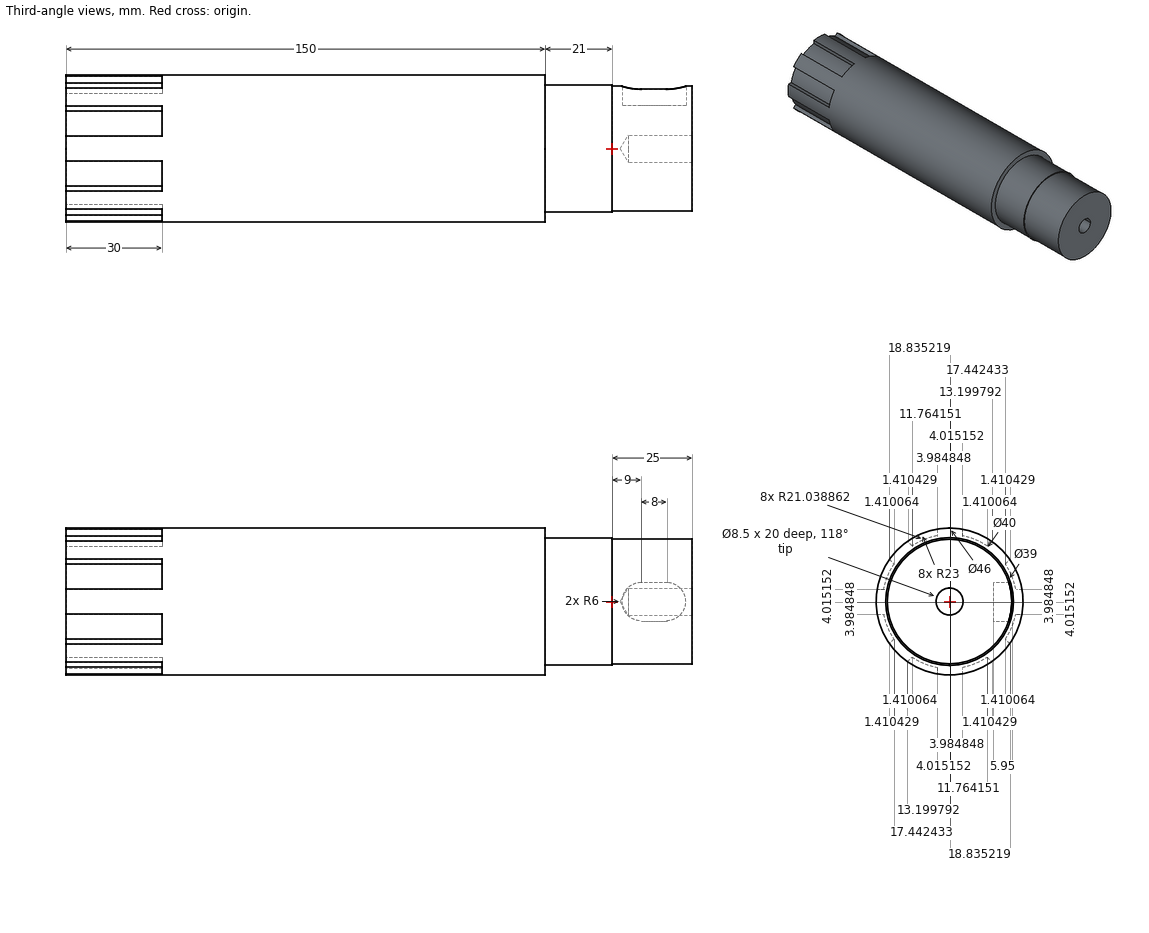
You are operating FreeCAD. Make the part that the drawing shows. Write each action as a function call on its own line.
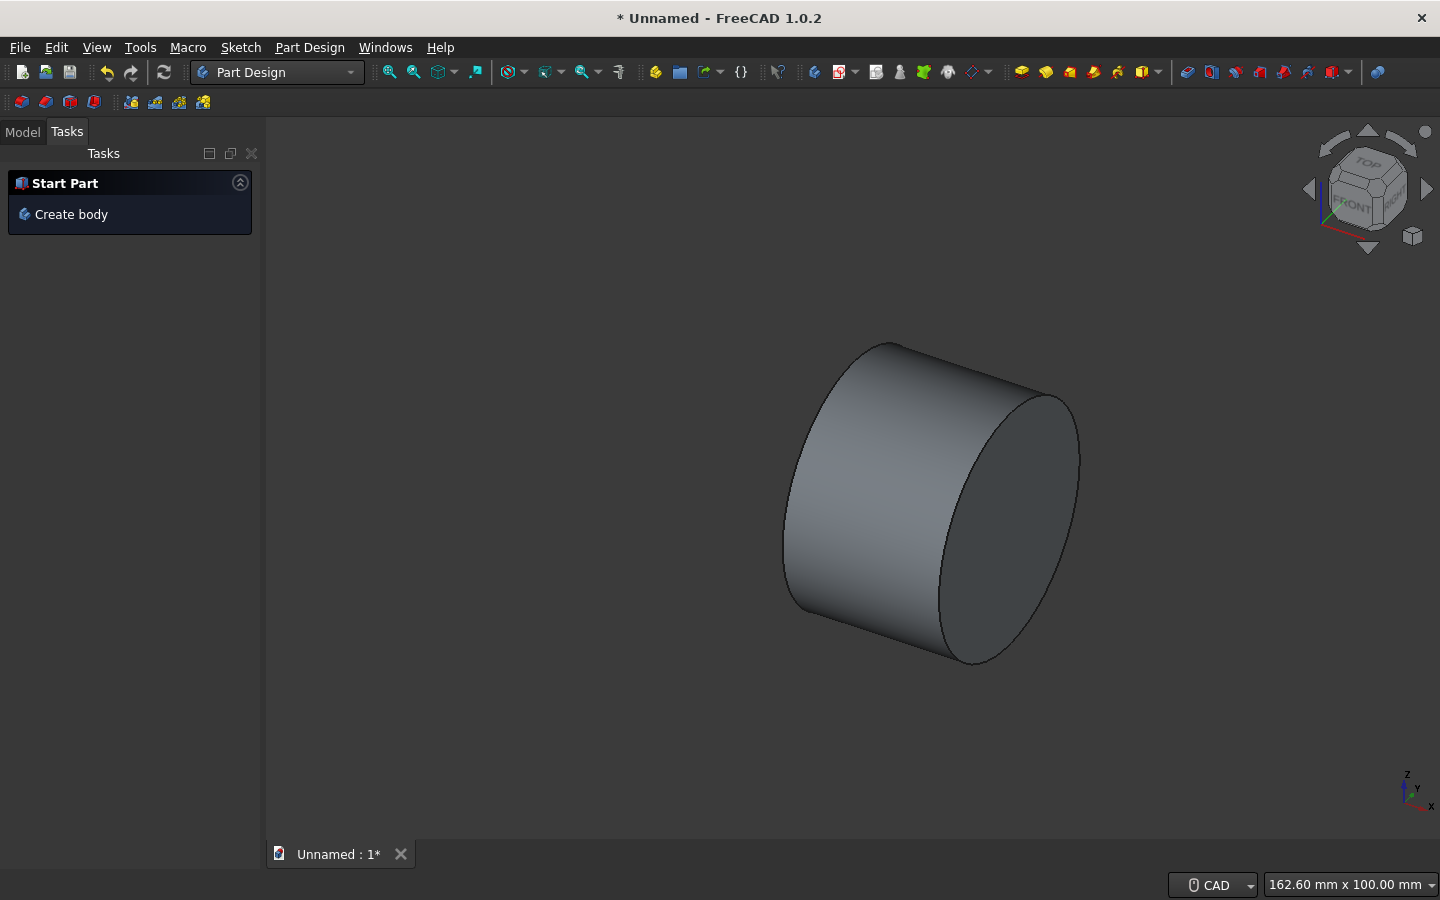
click(23, 131)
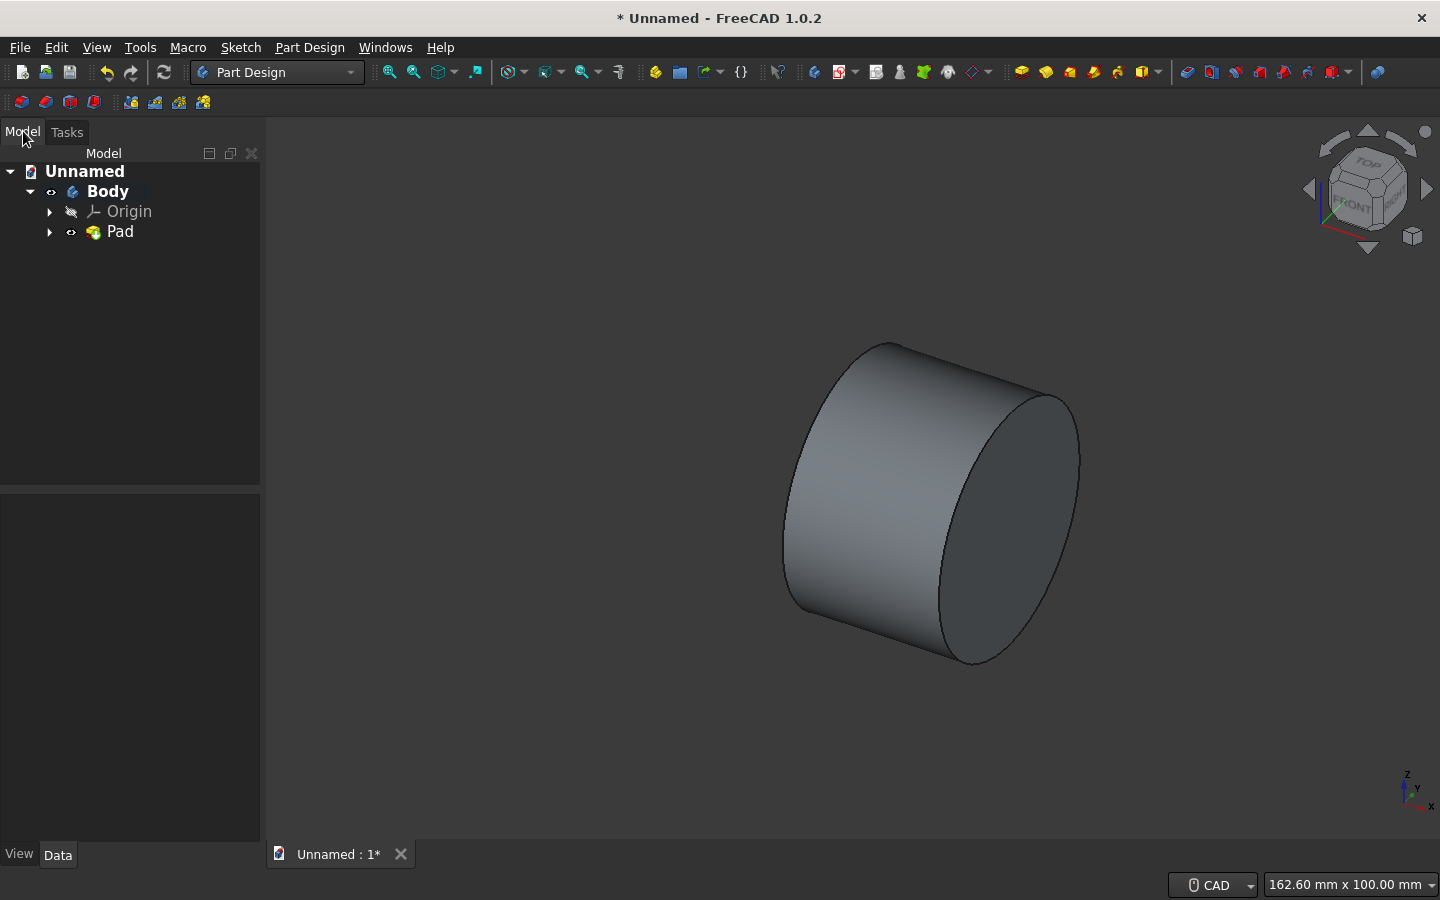
click(50, 212)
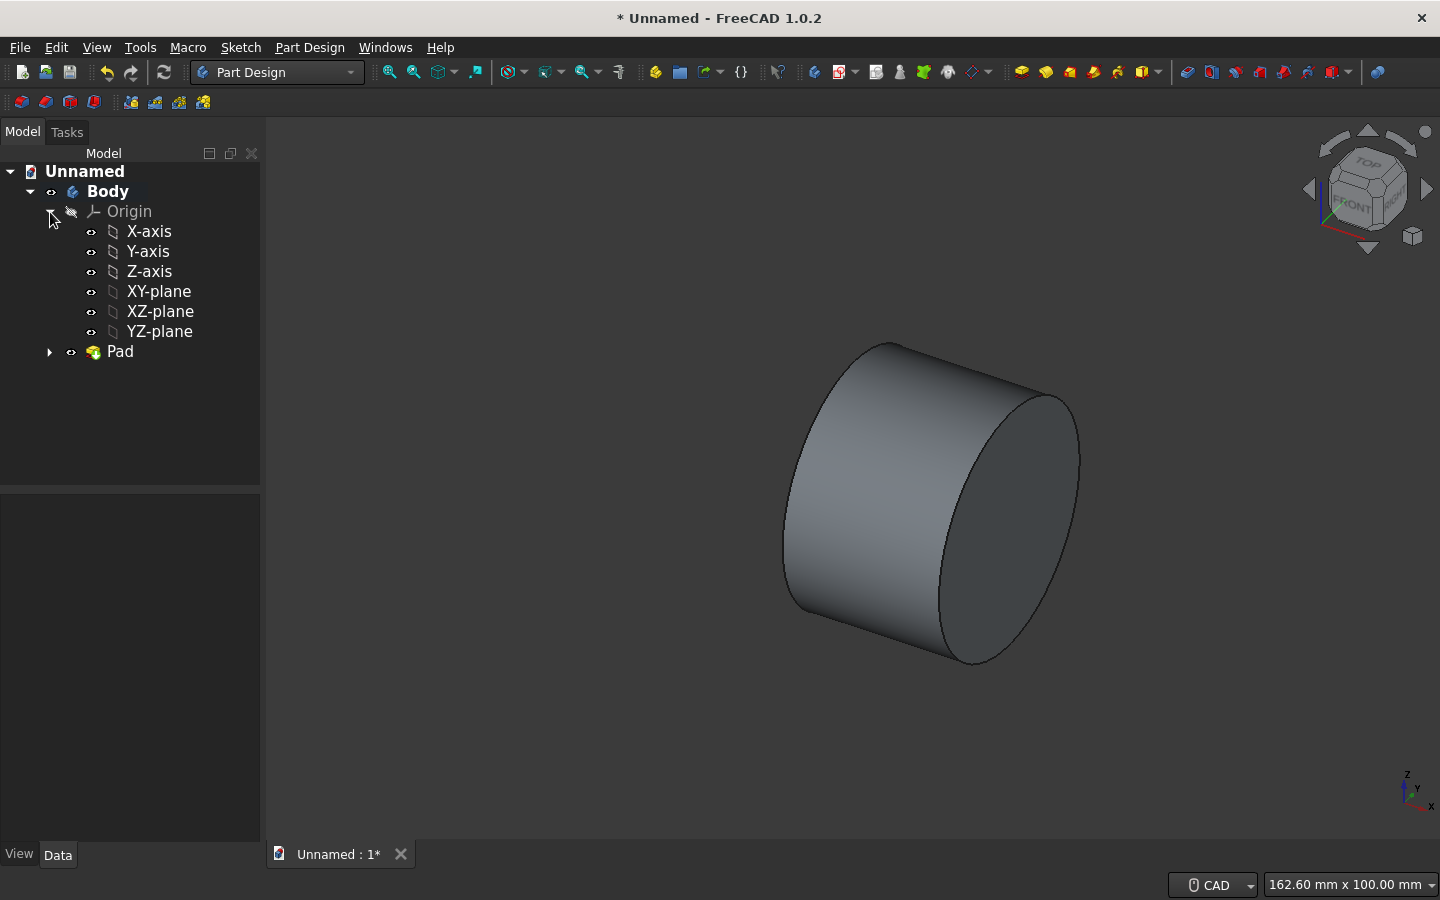
click(136, 312)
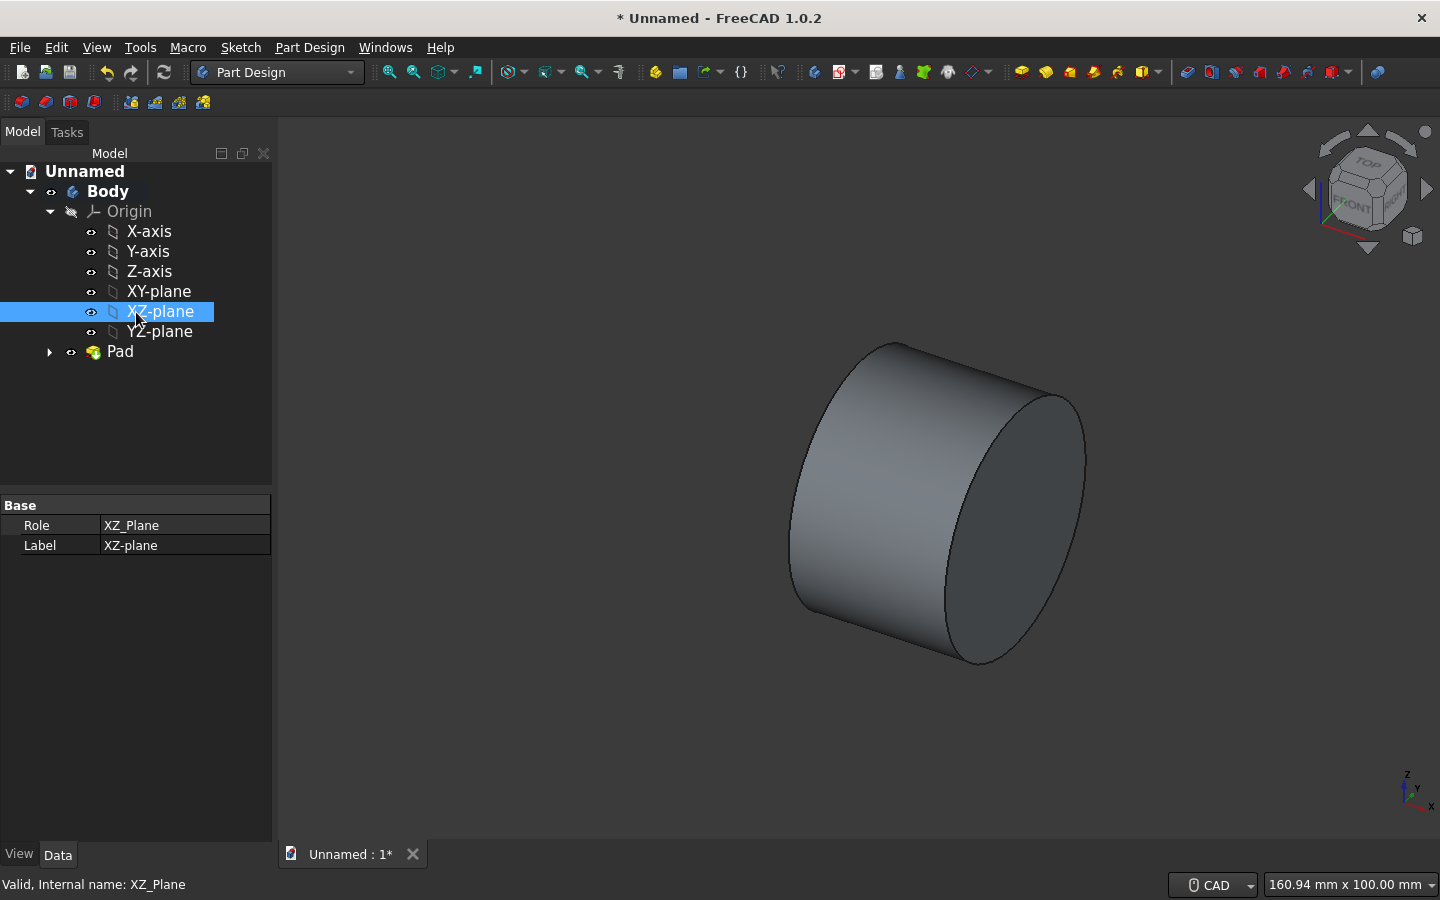
click(972, 72)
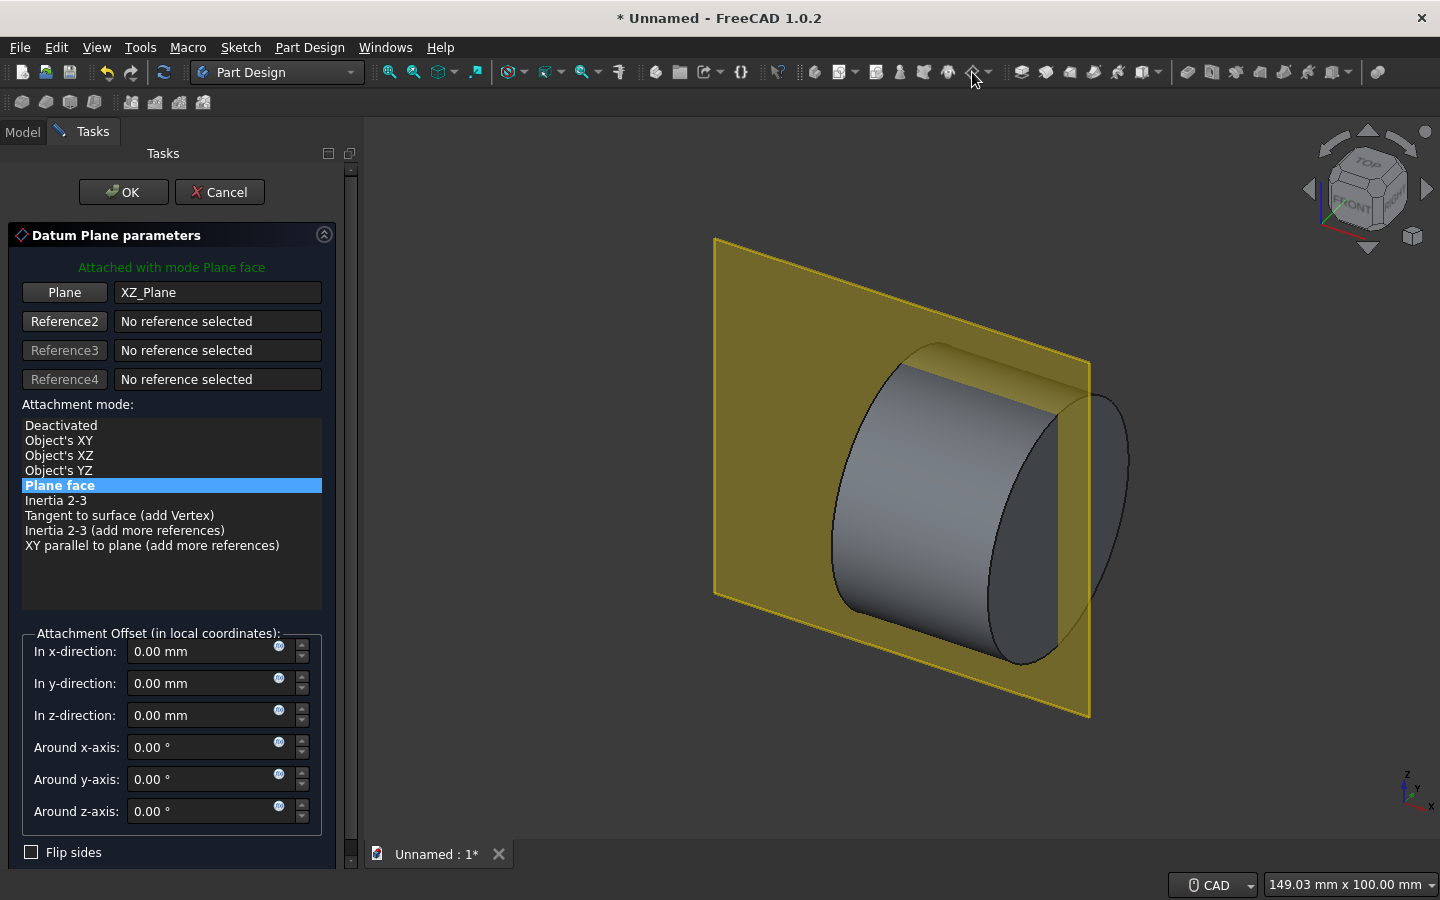
triple_click(210, 715)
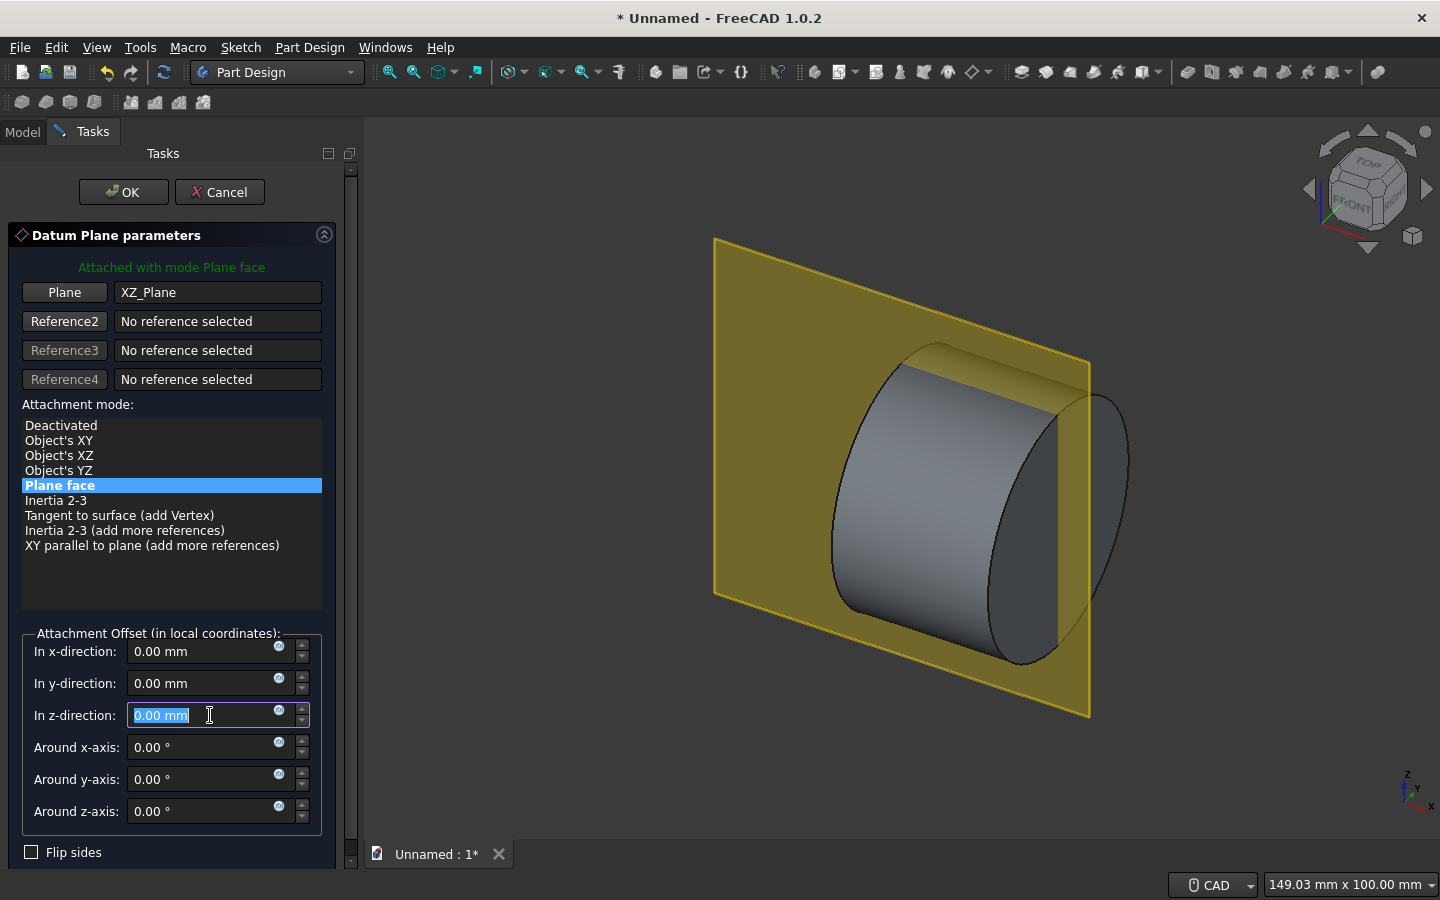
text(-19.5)
key(Tab)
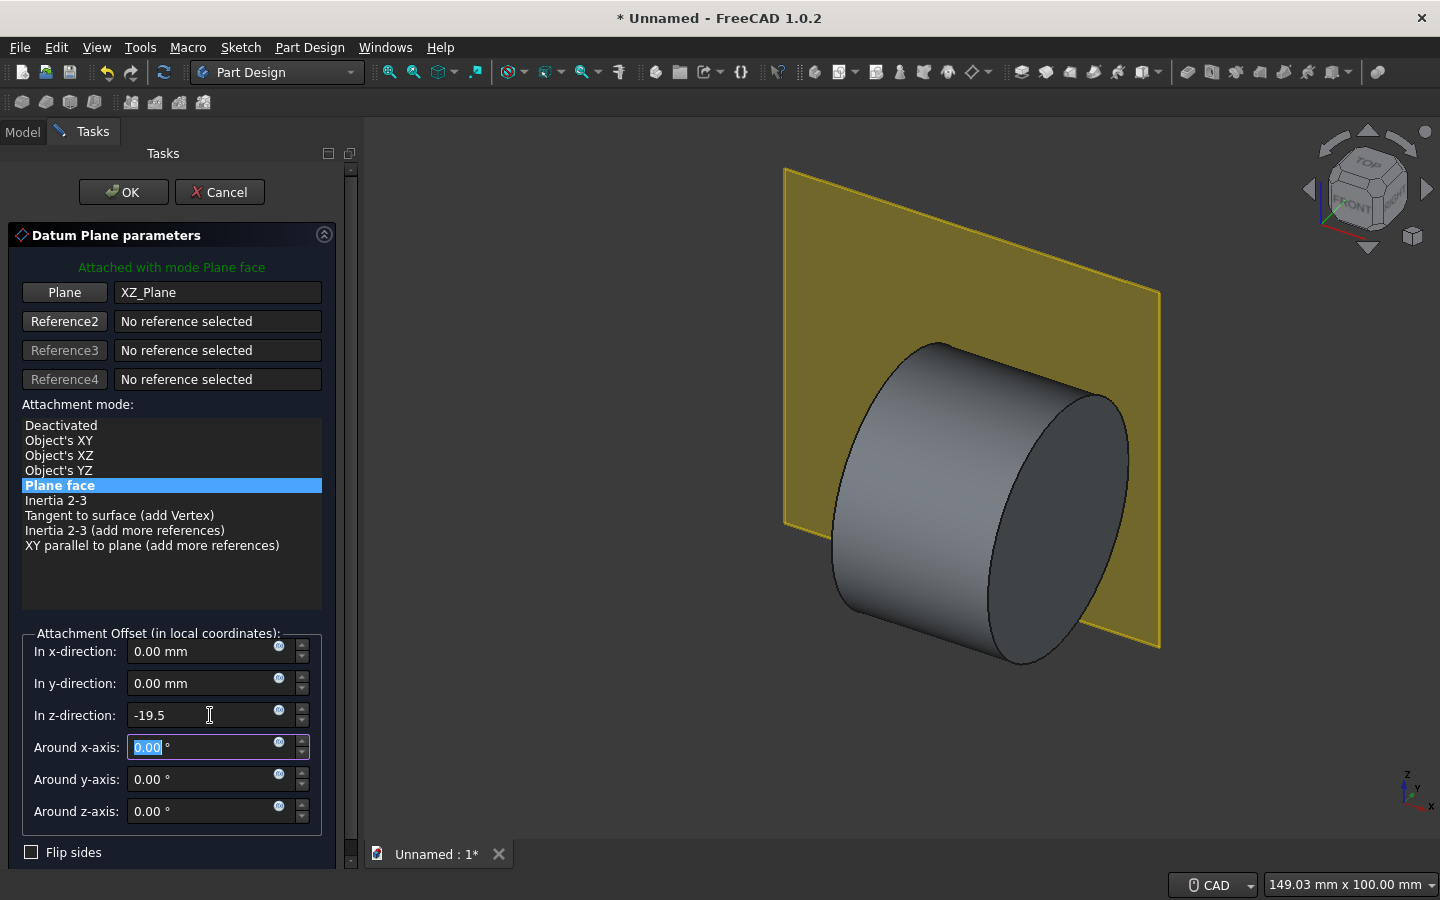
click(124, 192)